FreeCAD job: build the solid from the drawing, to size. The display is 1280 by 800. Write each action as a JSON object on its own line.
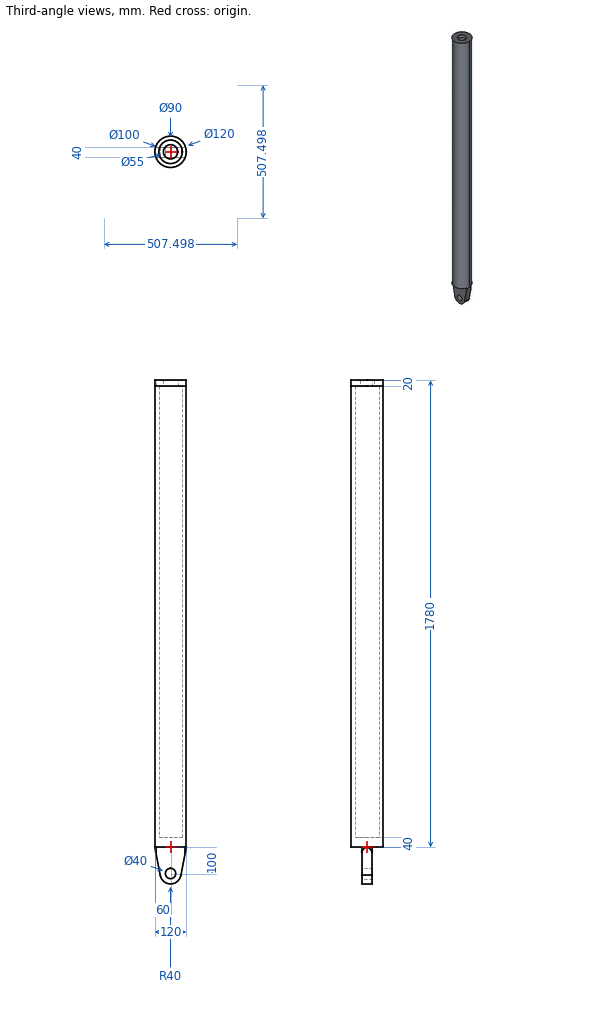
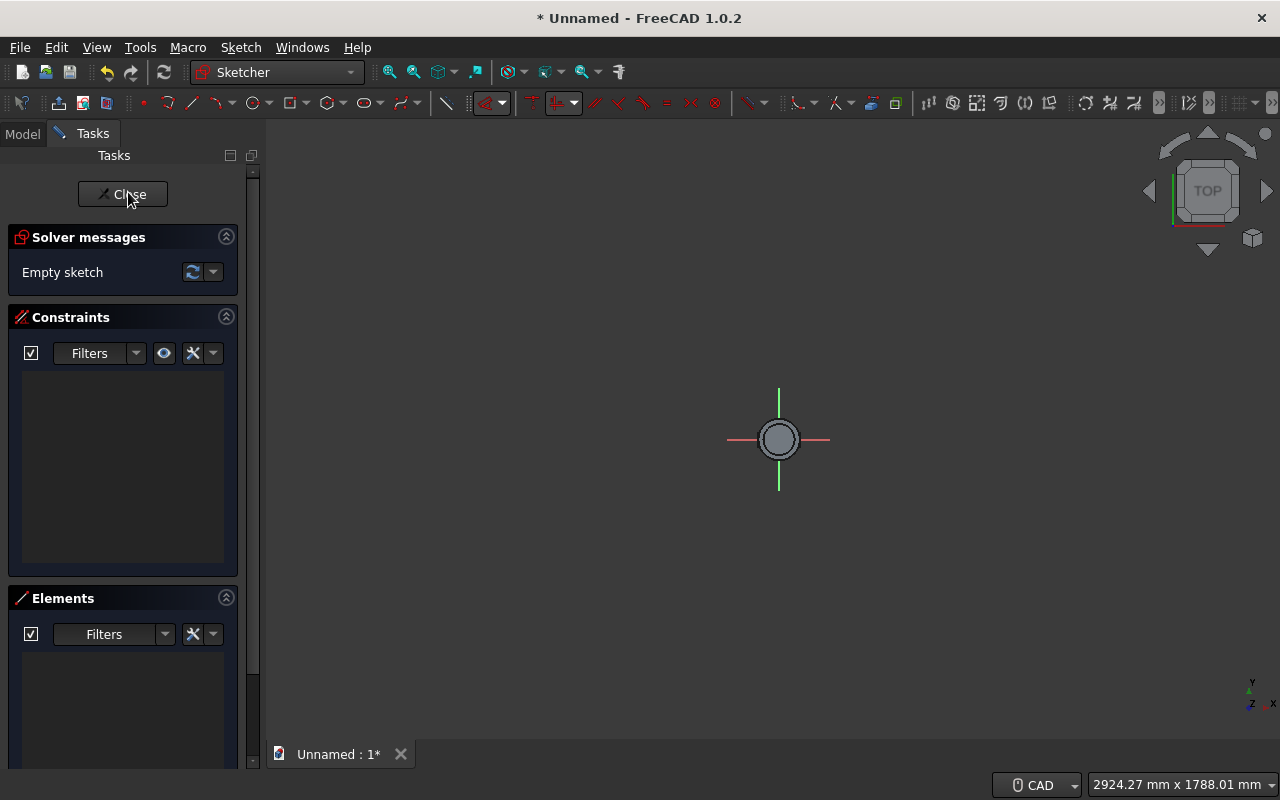
{"action": "key", "text": "q s"}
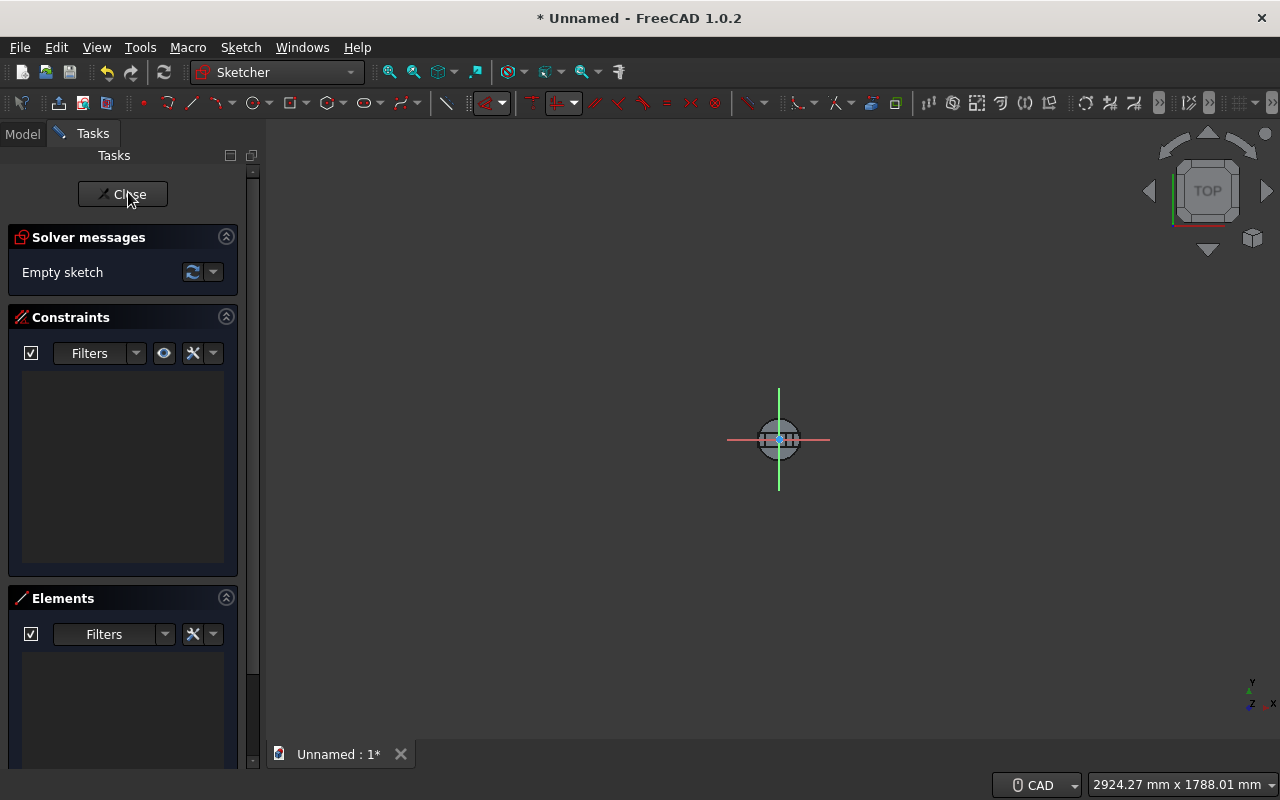
{"action": "scroll", "coordinate": [840, 448], "scroll_direction": "up", "scroll_amount": 4}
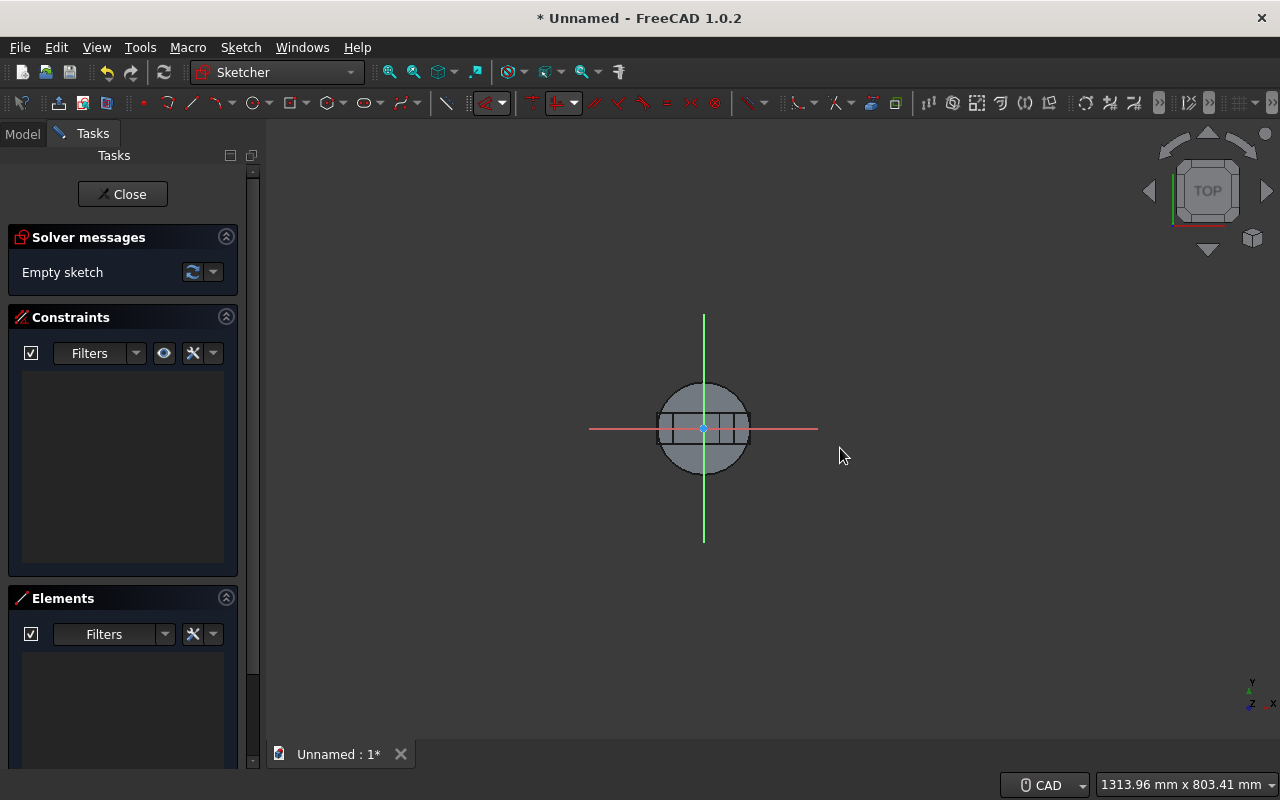
{"action": "key", "text": "g v"}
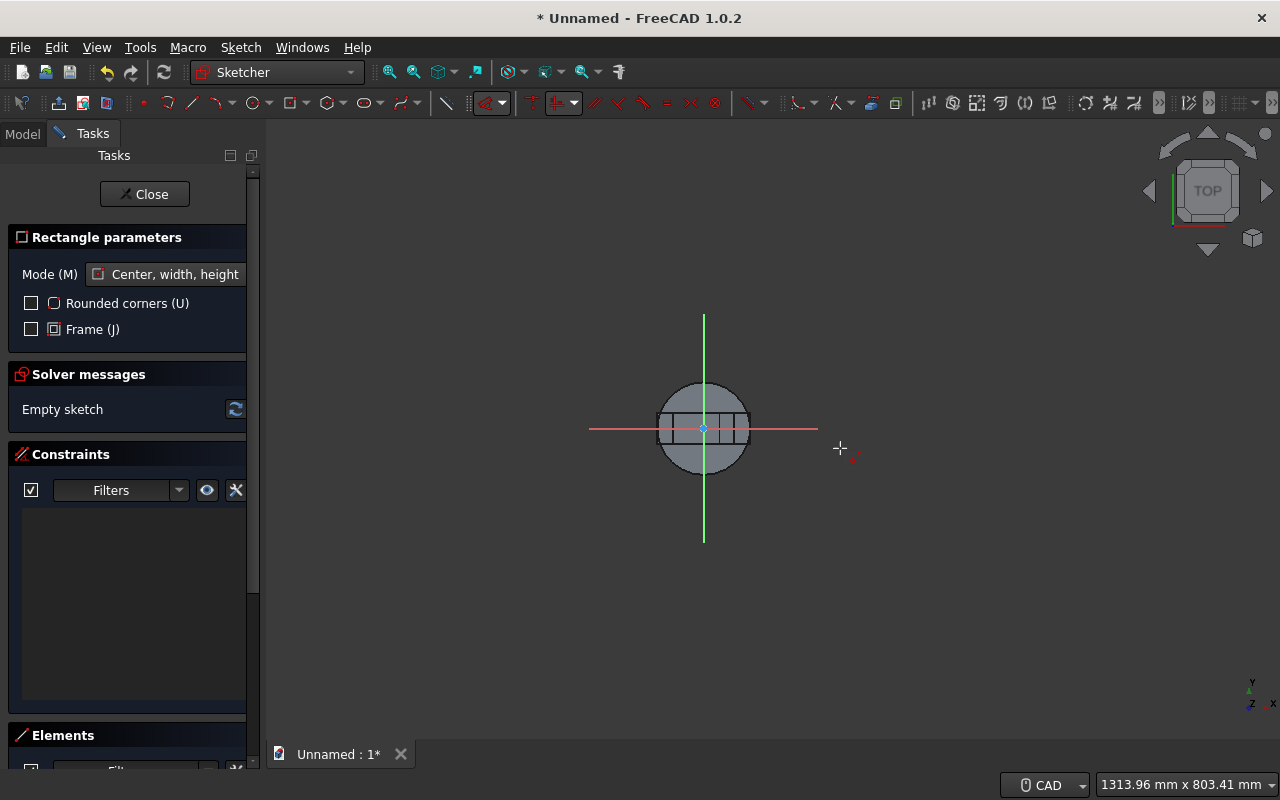
{"action": "left_click", "coordinate": [704, 429]}
{"action": "mouse_move", "coordinate": [900, 233]}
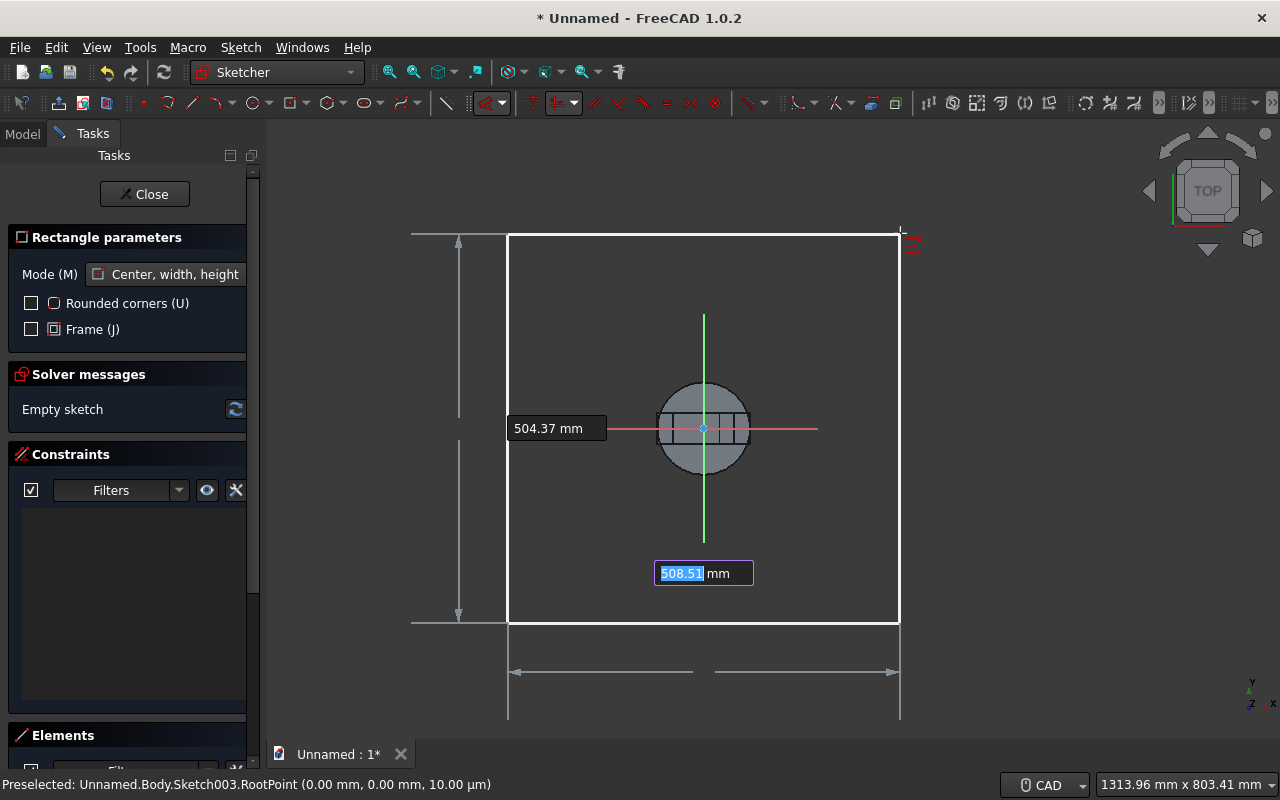
{"action": "type", "text": "507.498"}
{"action": "key", "text": "Tab"}
{"action": "type", "text": "507.498"}
{"action": "key", "text": "Return"}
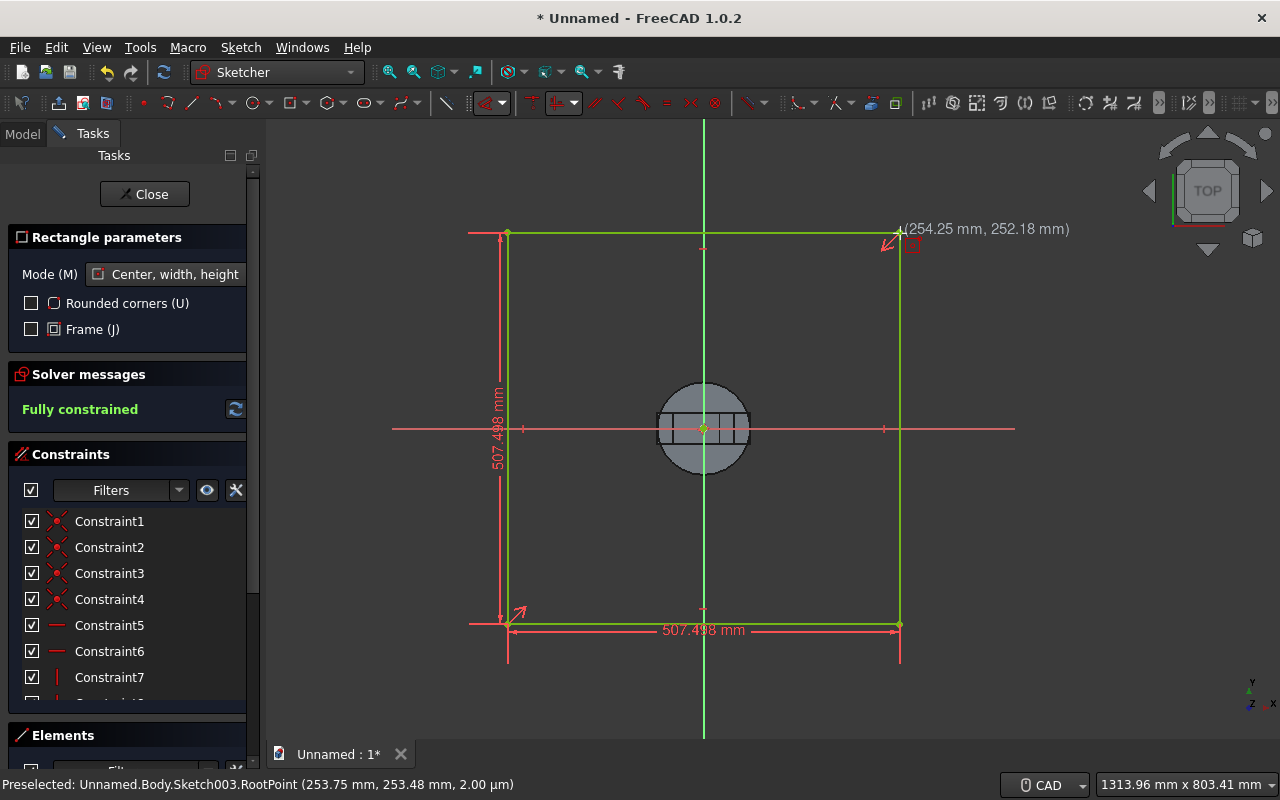
{"action": "key", "text": "g c"}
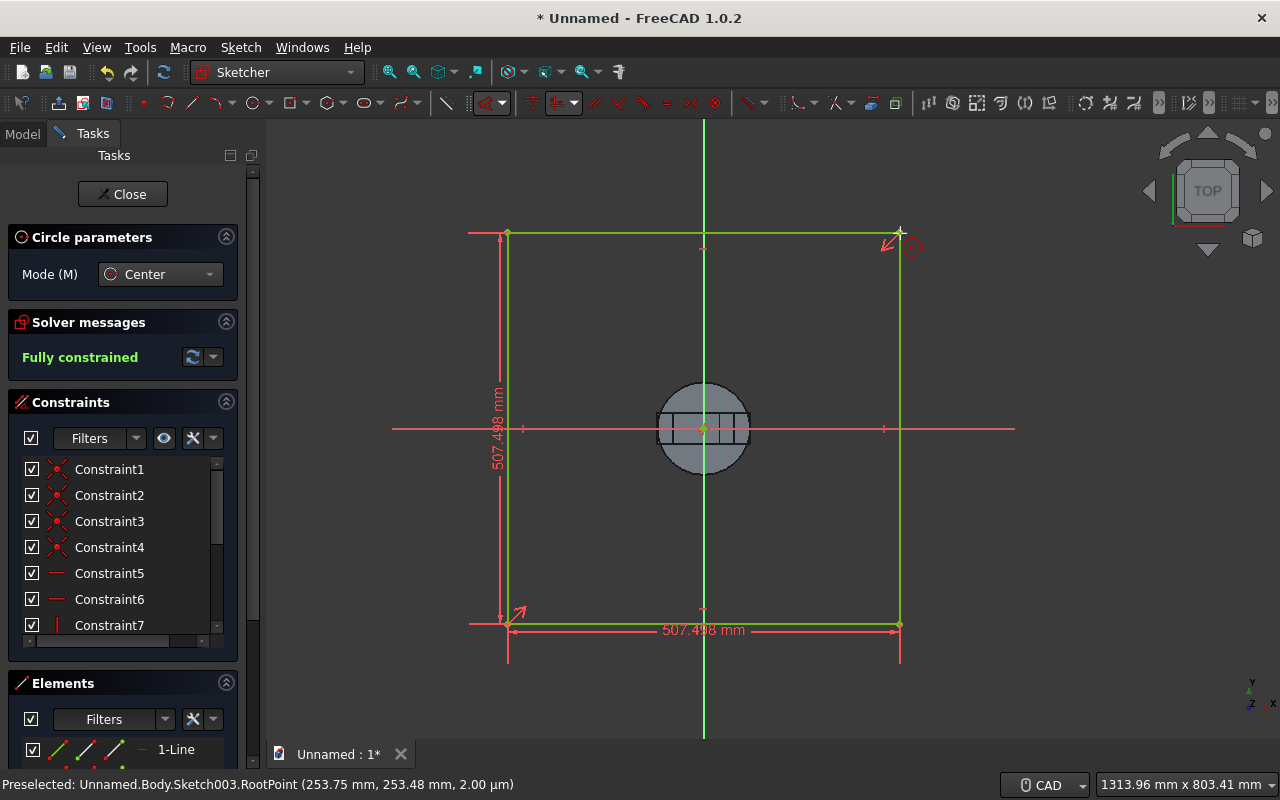
{"action": "left_click", "coordinate": [704, 429]}
{"action": "mouse_move", "coordinate": [737, 396]}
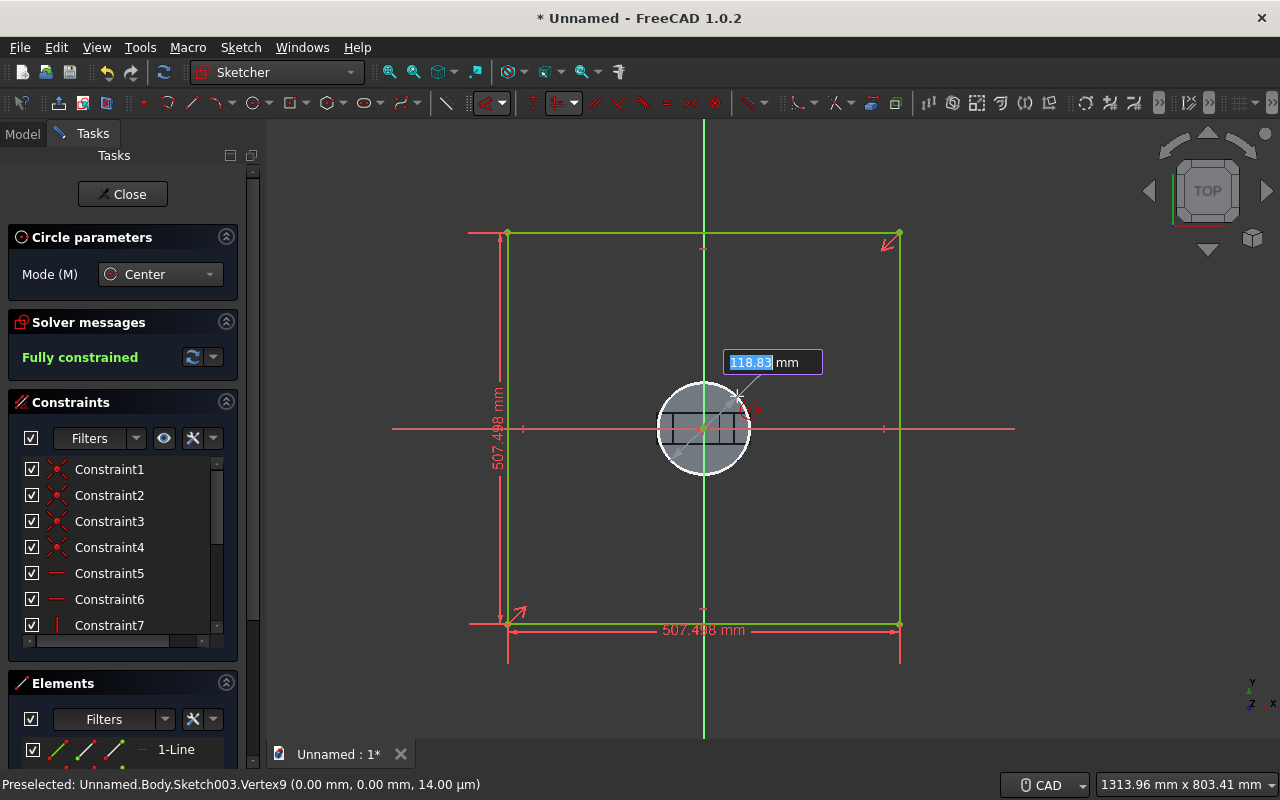
{"action": "type", "text": "120"}
{"action": "key", "text": "Return"}
{"action": "key", "text": "Escape"}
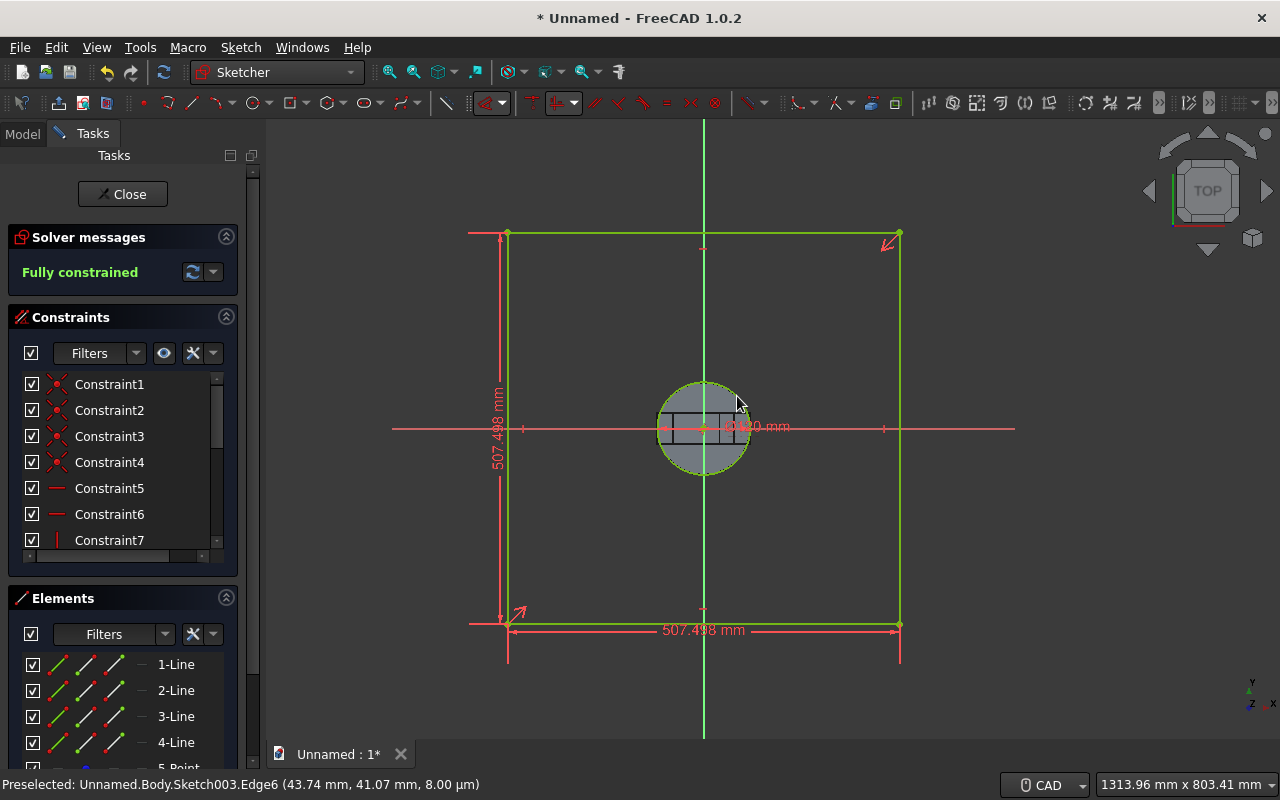
{"action": "left_click", "coordinate": [123, 194]}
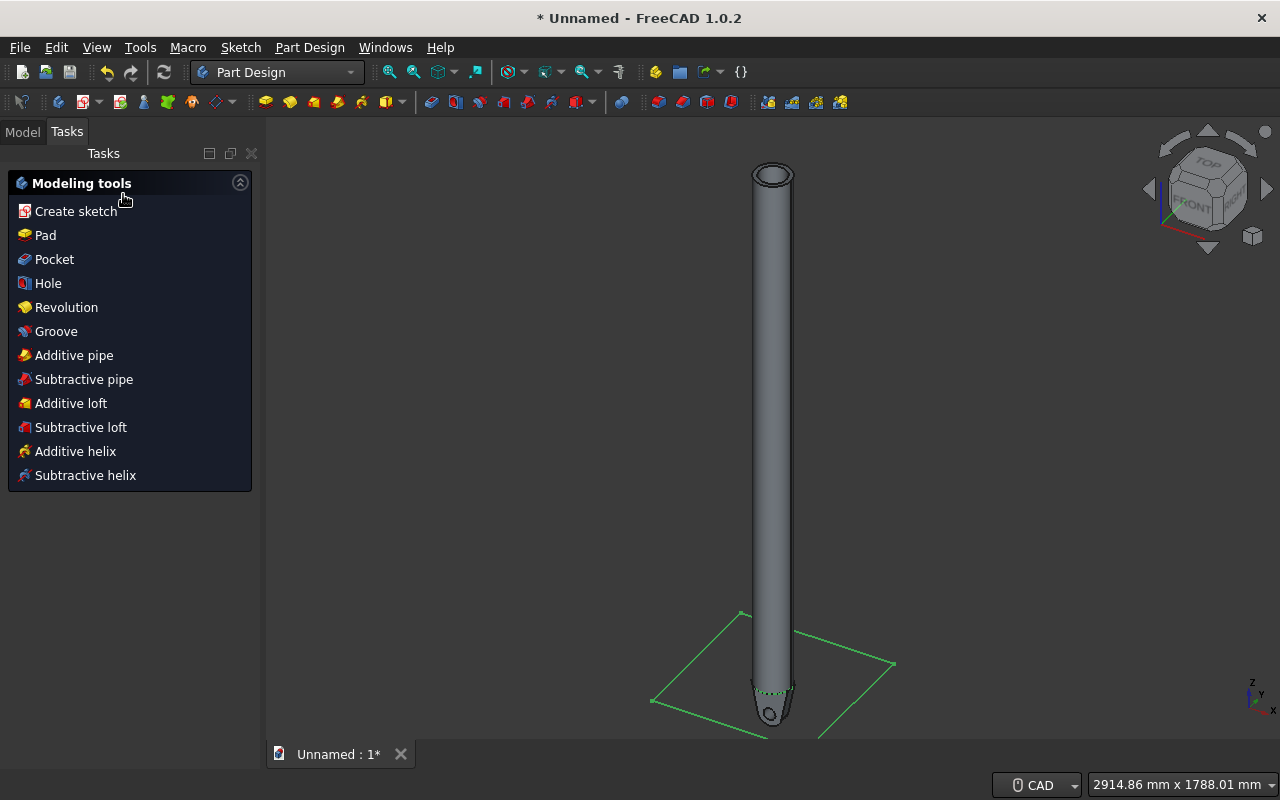
{"action": "left_click", "coordinate": [432, 102]}